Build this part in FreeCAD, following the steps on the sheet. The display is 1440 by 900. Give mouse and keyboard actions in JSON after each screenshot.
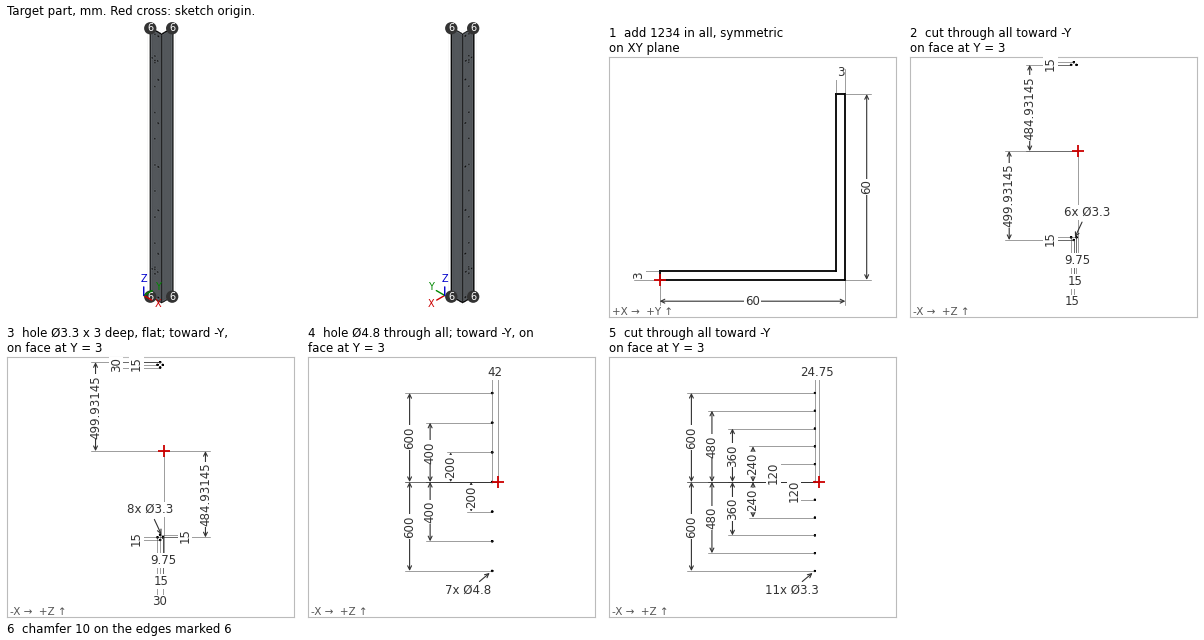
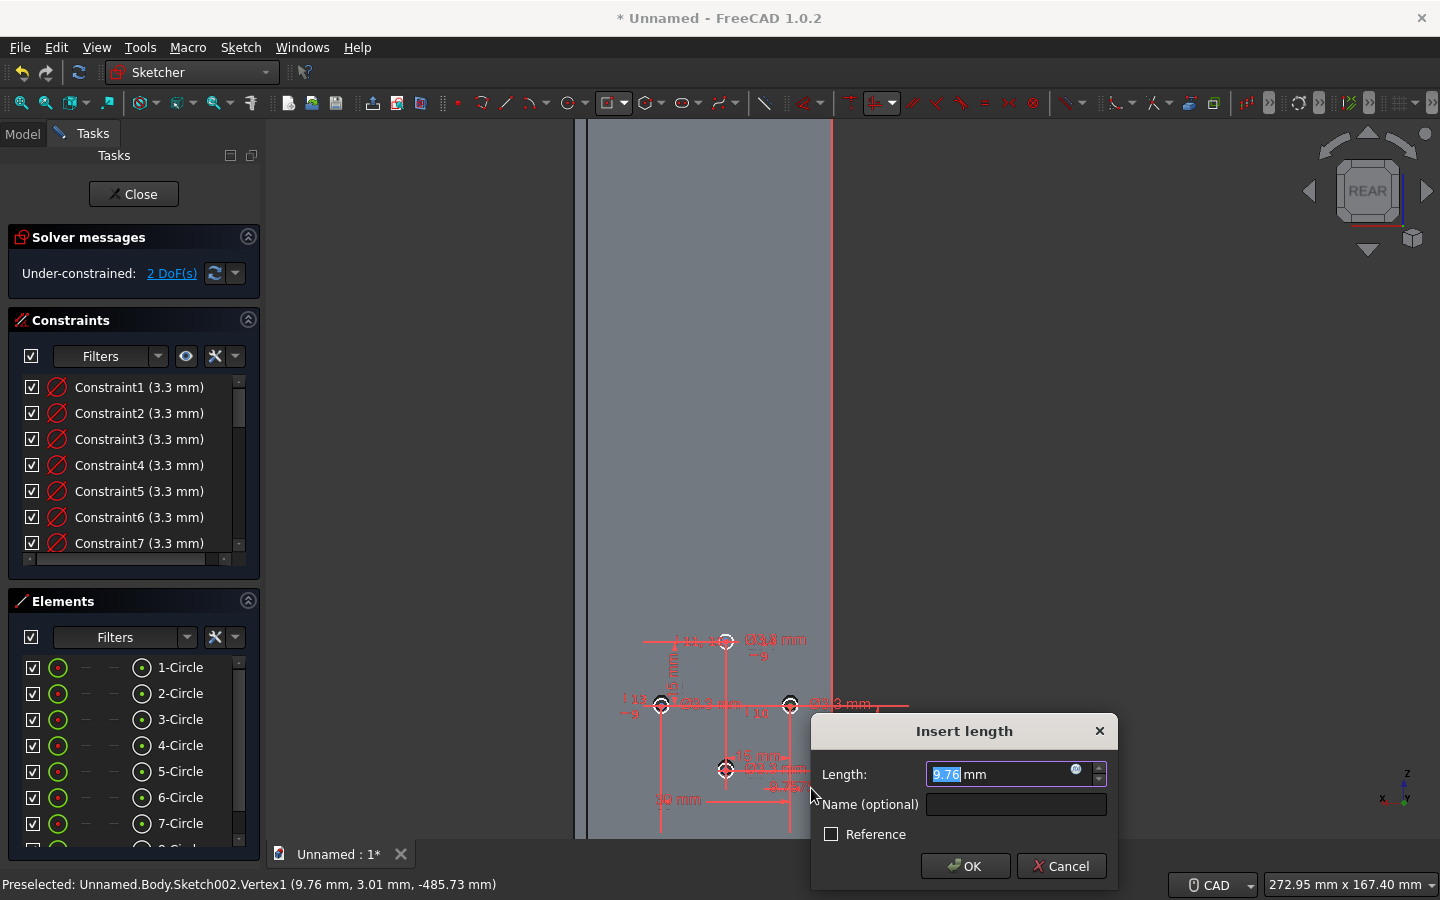
{"action": "type", "text": "9.75"}
{"action": "key", "text": "Return"}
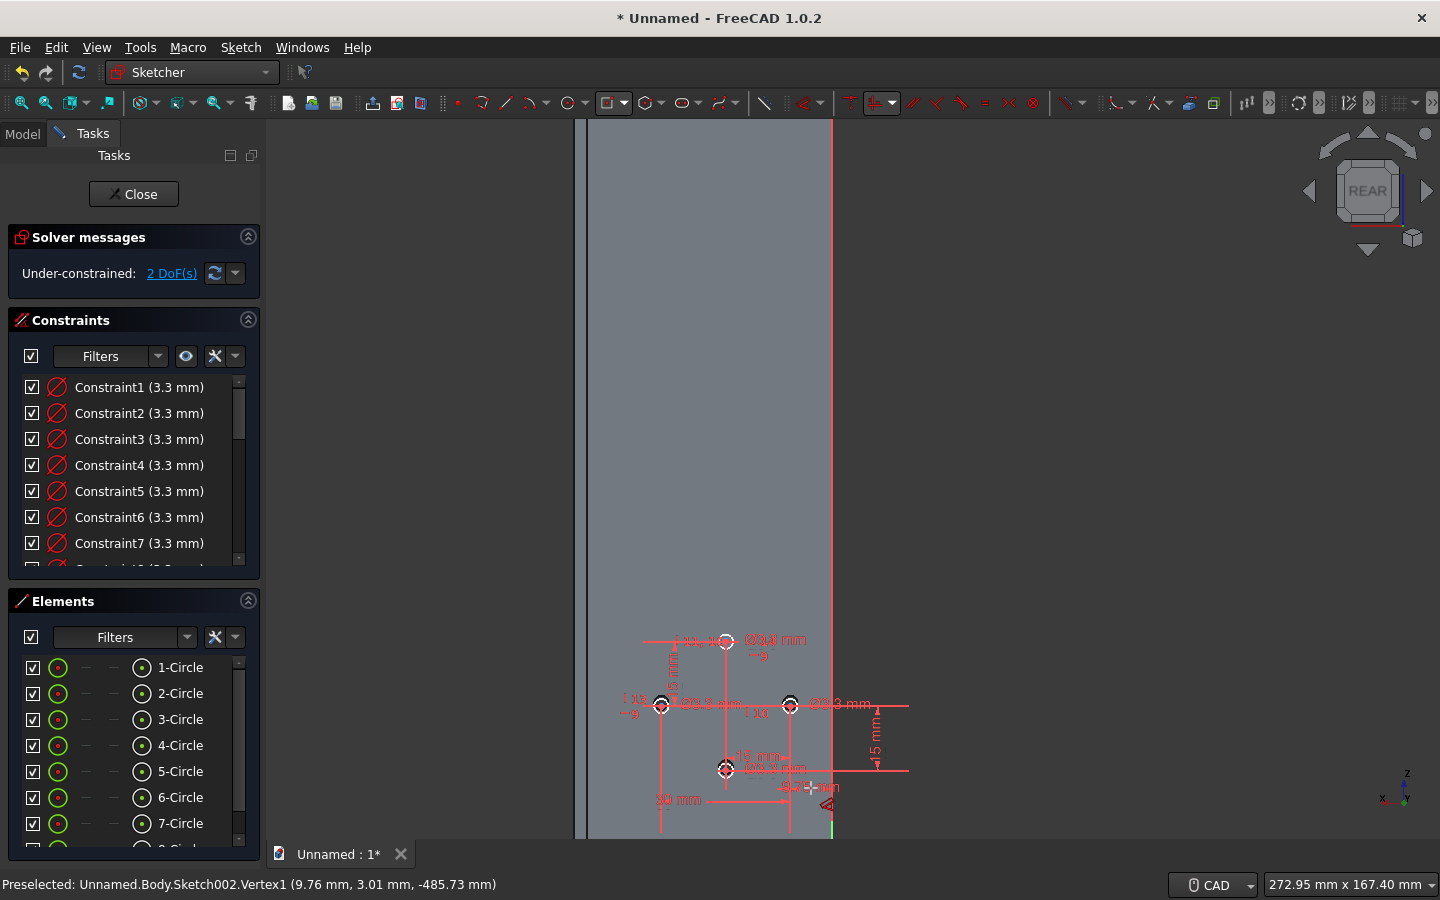
{"action": "scroll", "coordinate": [790, 711], "scroll_direction": "down", "scroll_amount": 11}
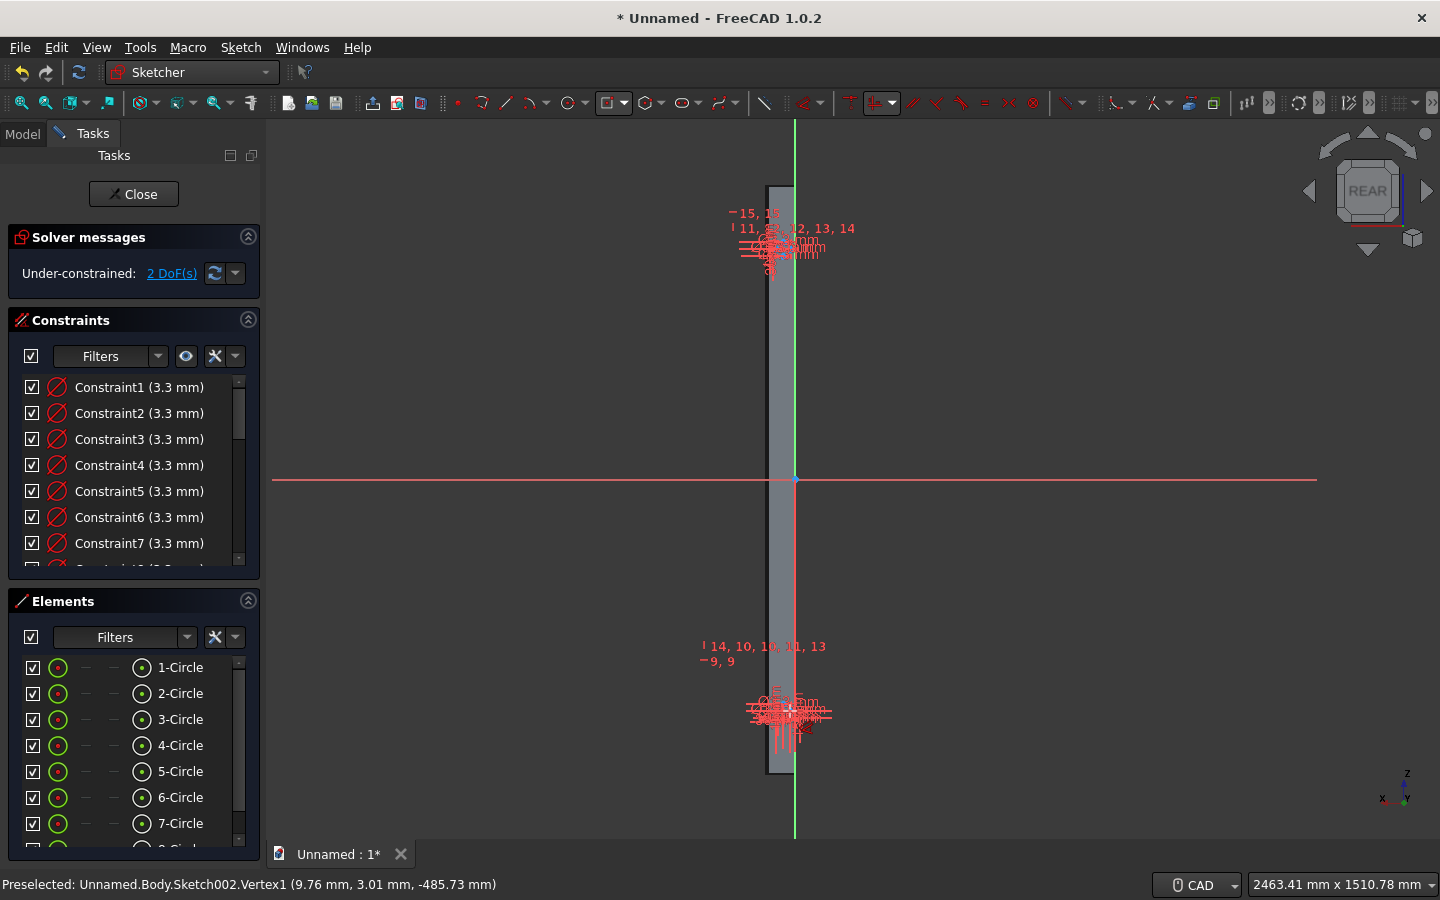
{"action": "left_click", "coordinate": [790, 711]}
{"action": "left_click", "coordinate": [829, 595]}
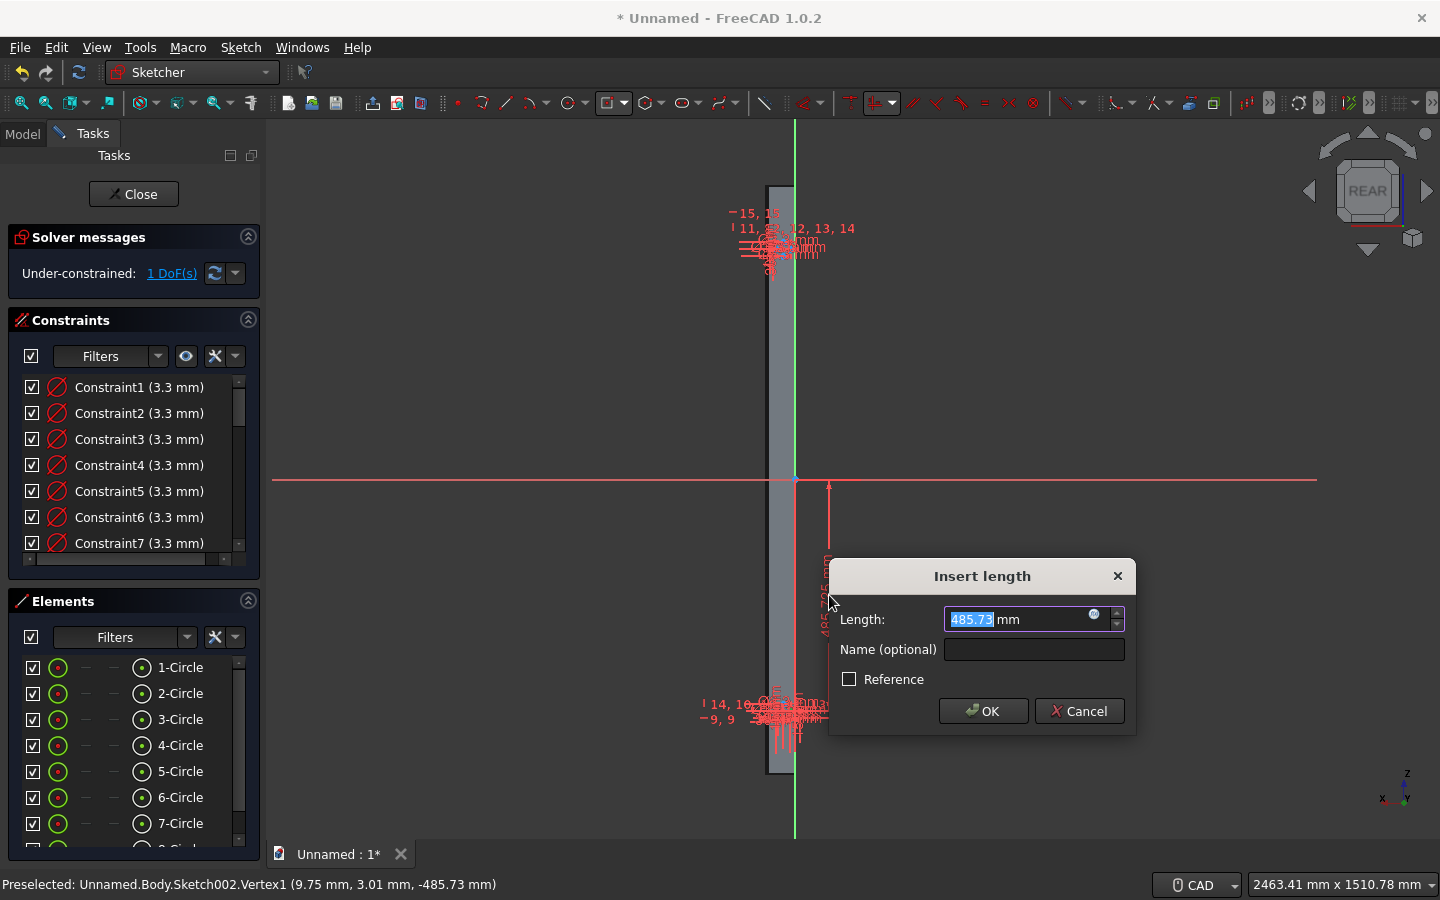
{"action": "type", "text": "484.93145"}
{"action": "key", "text": "Return"}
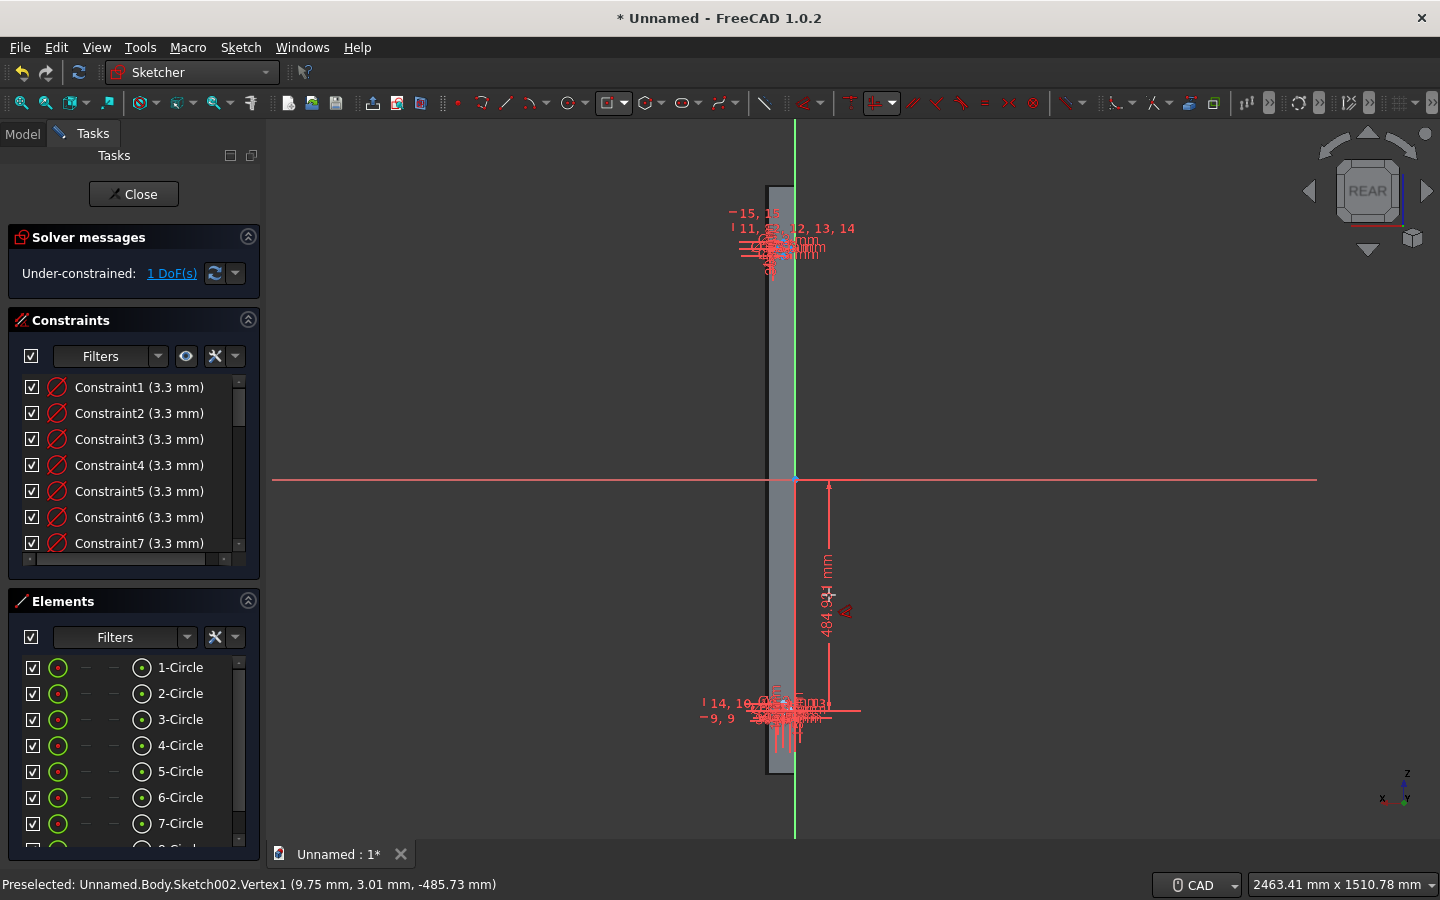
{"action": "left_click", "coordinate": [783, 242]}
{"action": "left_click", "coordinate": [829, 361]}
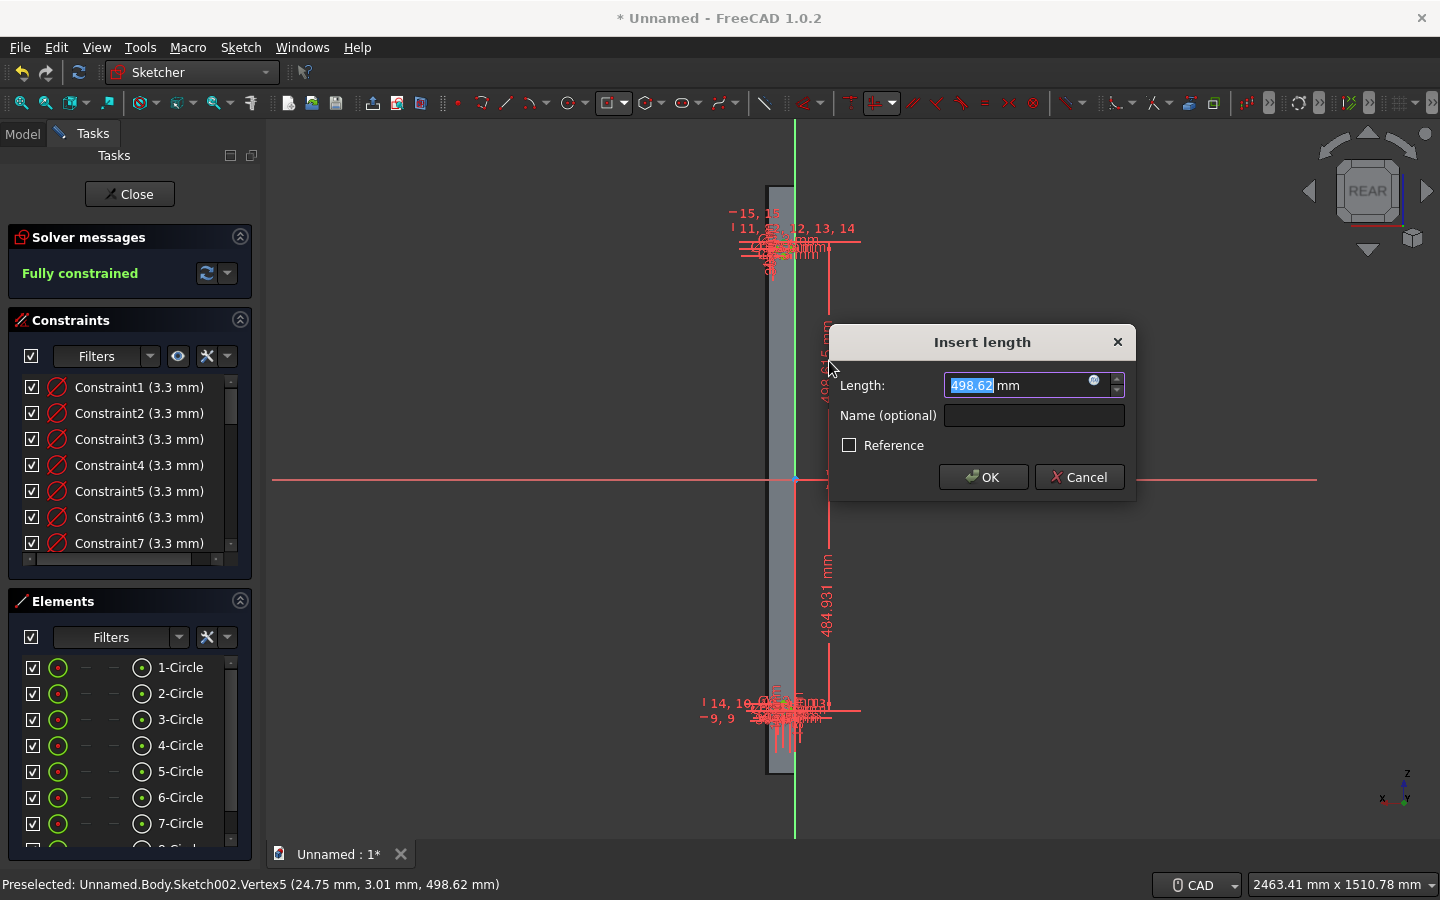
{"action": "type", "text": "499.93145"}
{"action": "key", "text": "Return"}
{"action": "key", "text": "Escape"}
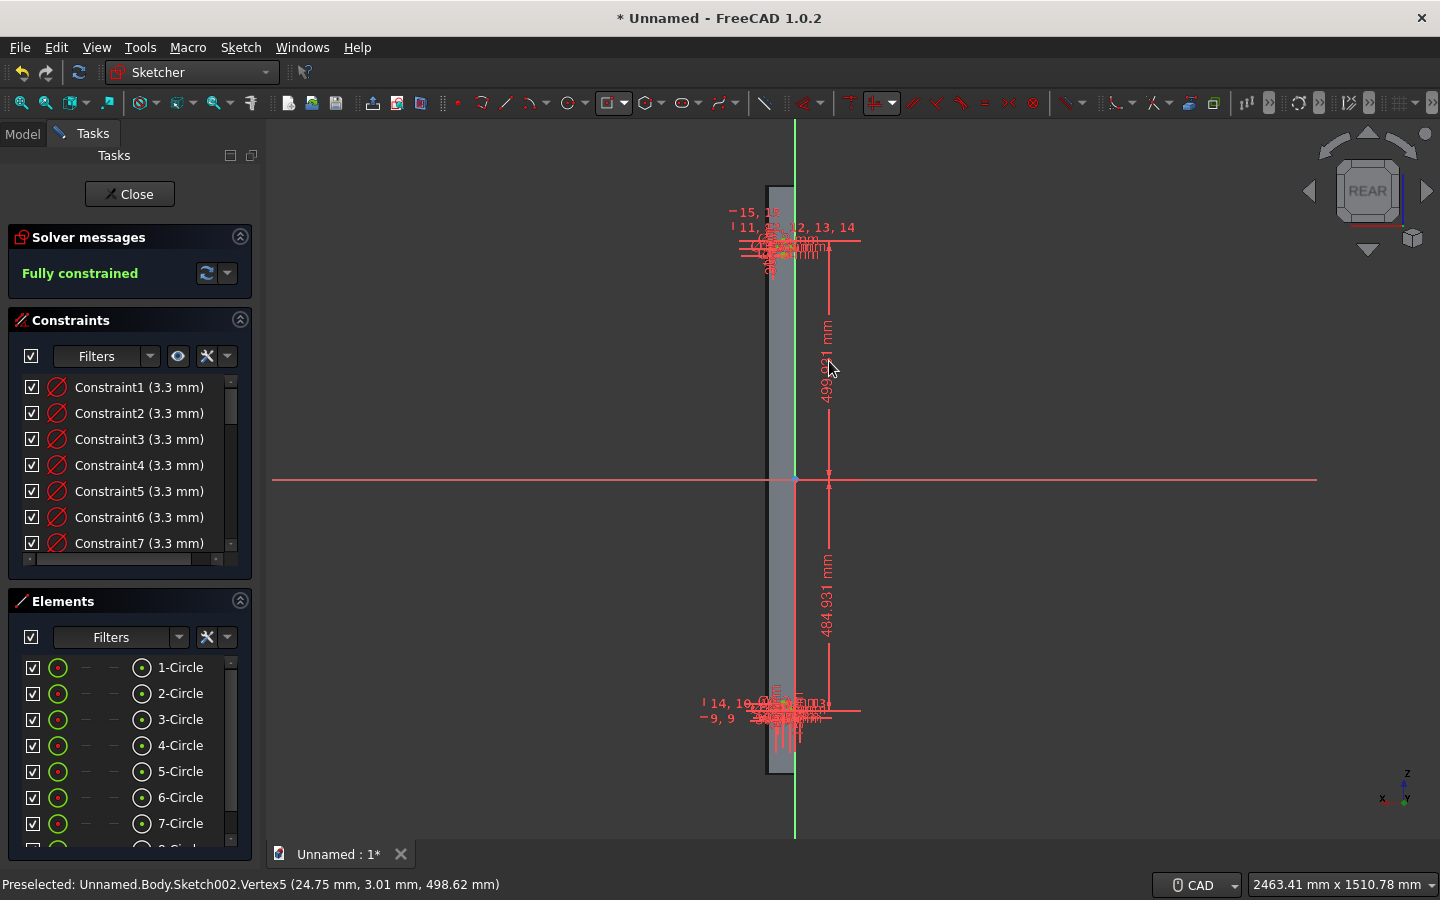
{"action": "left_click", "coordinate": [130, 194]}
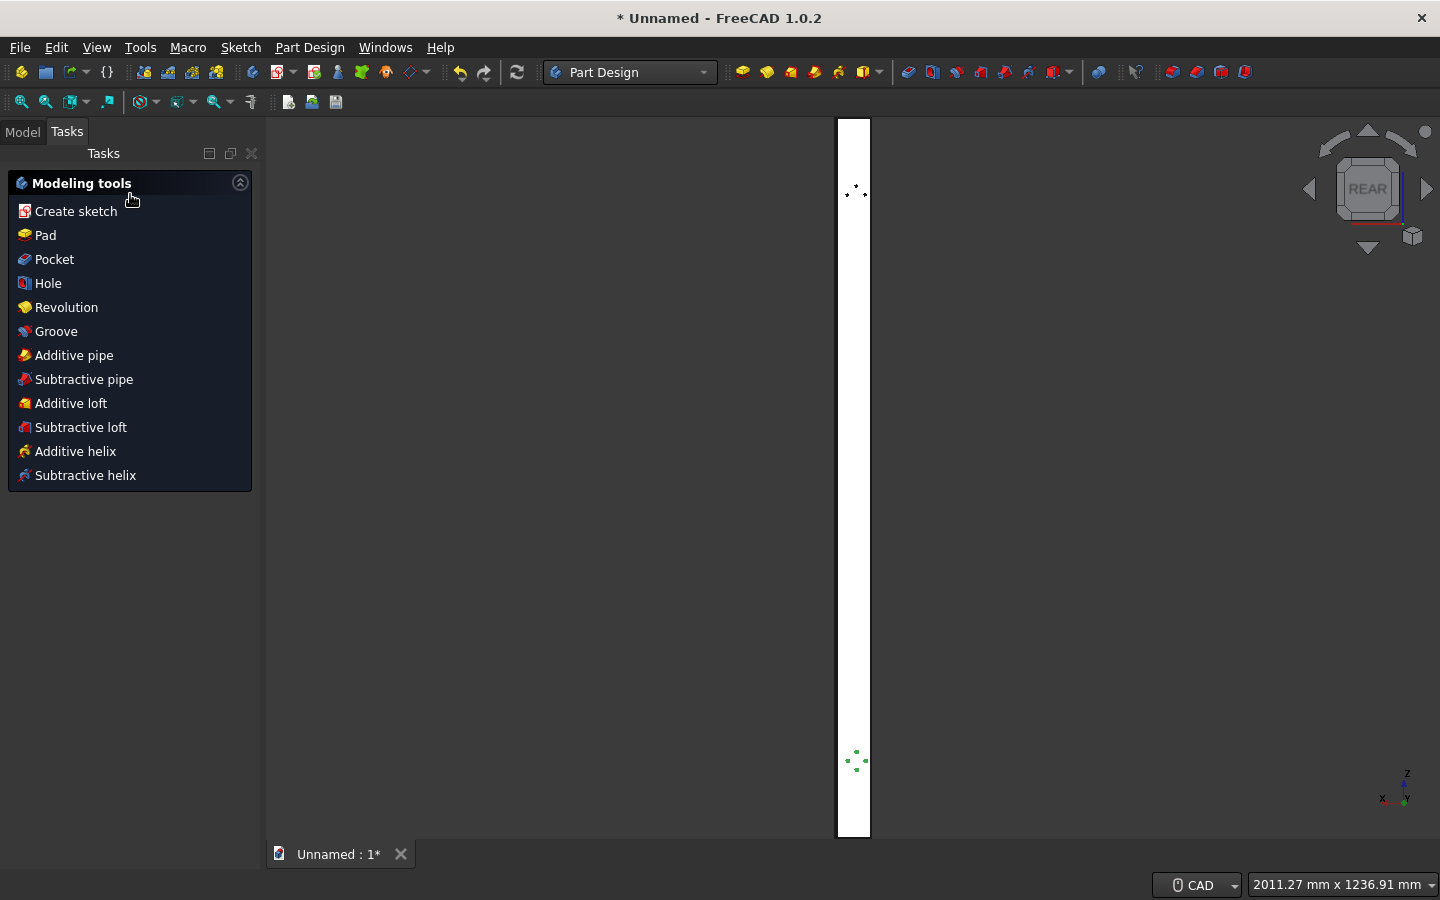
{"action": "left_click", "coordinate": [934, 72]}